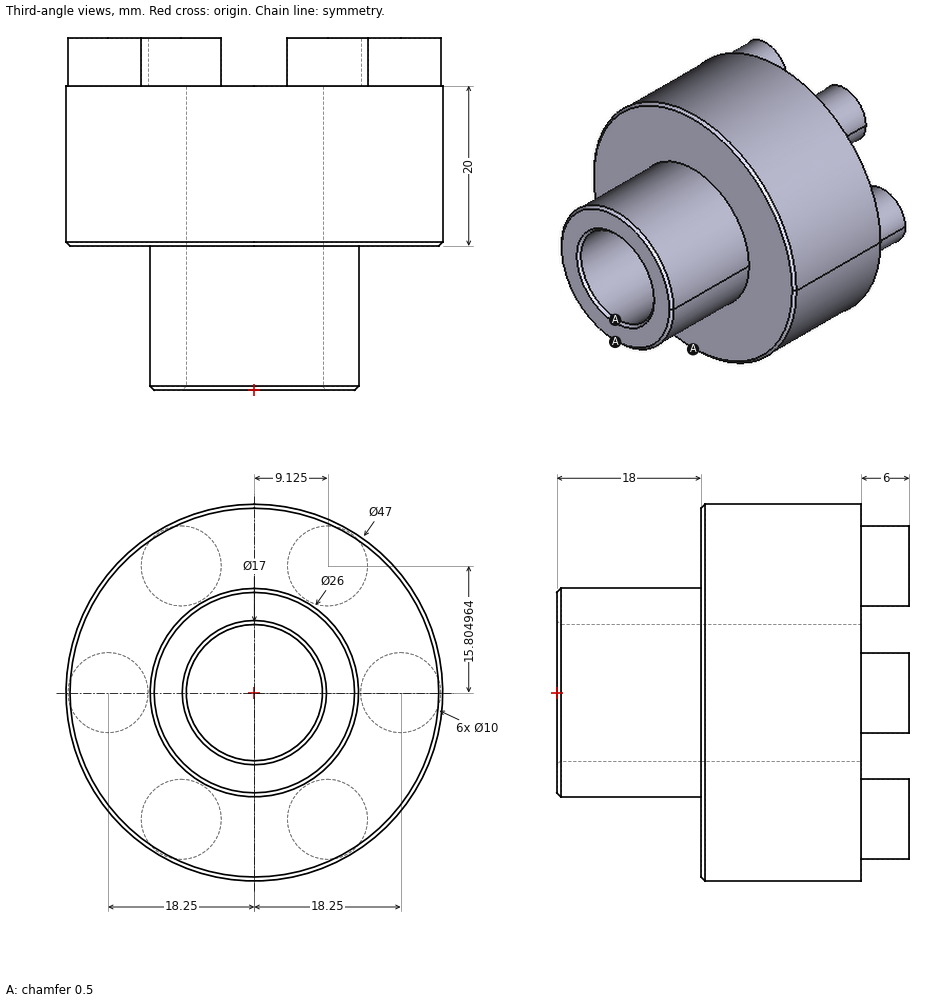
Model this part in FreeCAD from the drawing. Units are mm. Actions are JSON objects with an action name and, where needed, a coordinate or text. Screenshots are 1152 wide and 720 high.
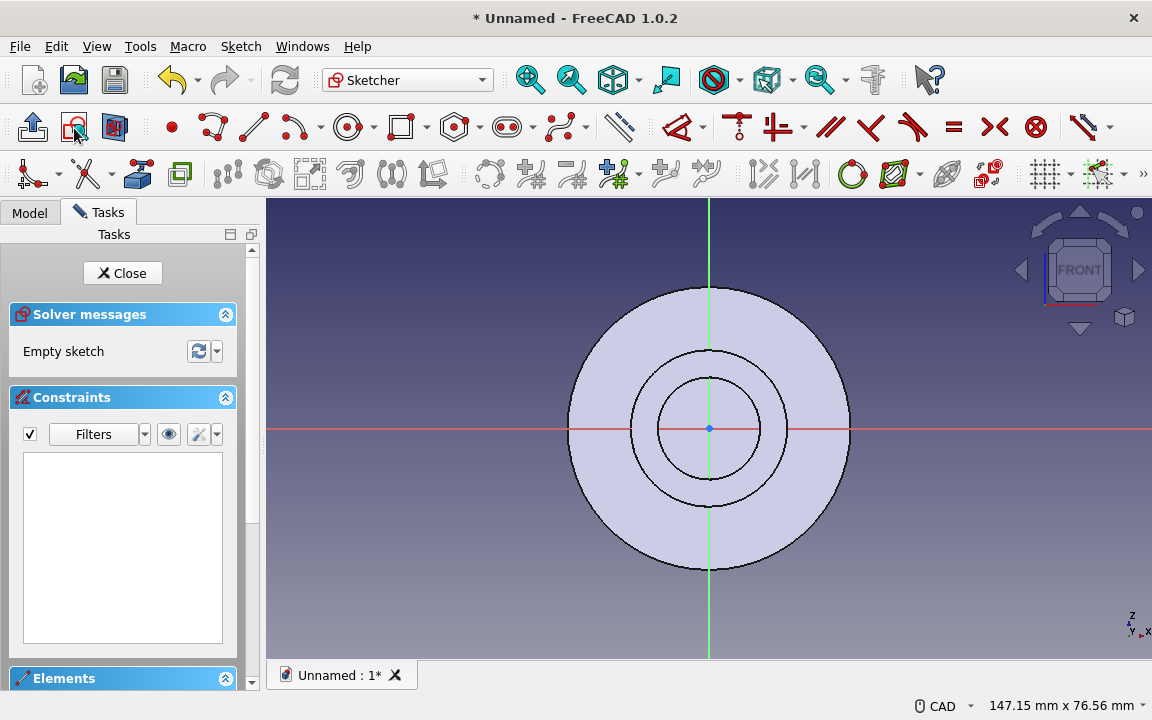
{"action": "left_click", "coordinate": [115, 128]}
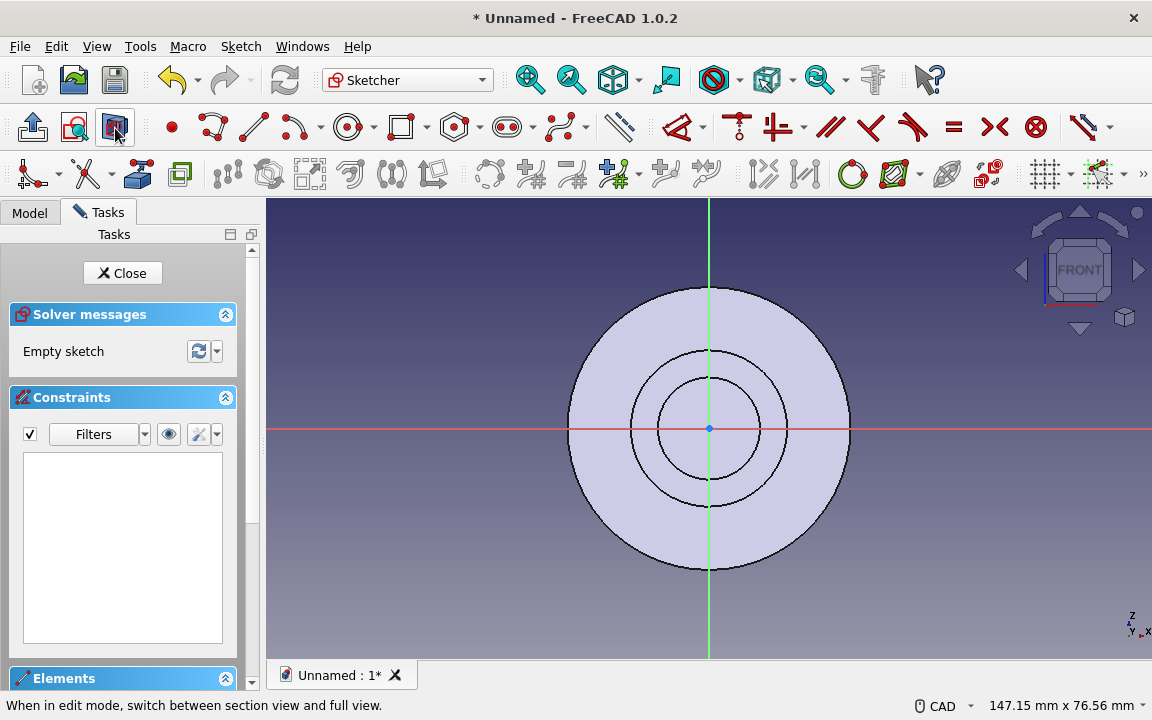
{"action": "scroll", "coordinate": [749, 429], "scroll_direction": "up", "scroll_amount": 5}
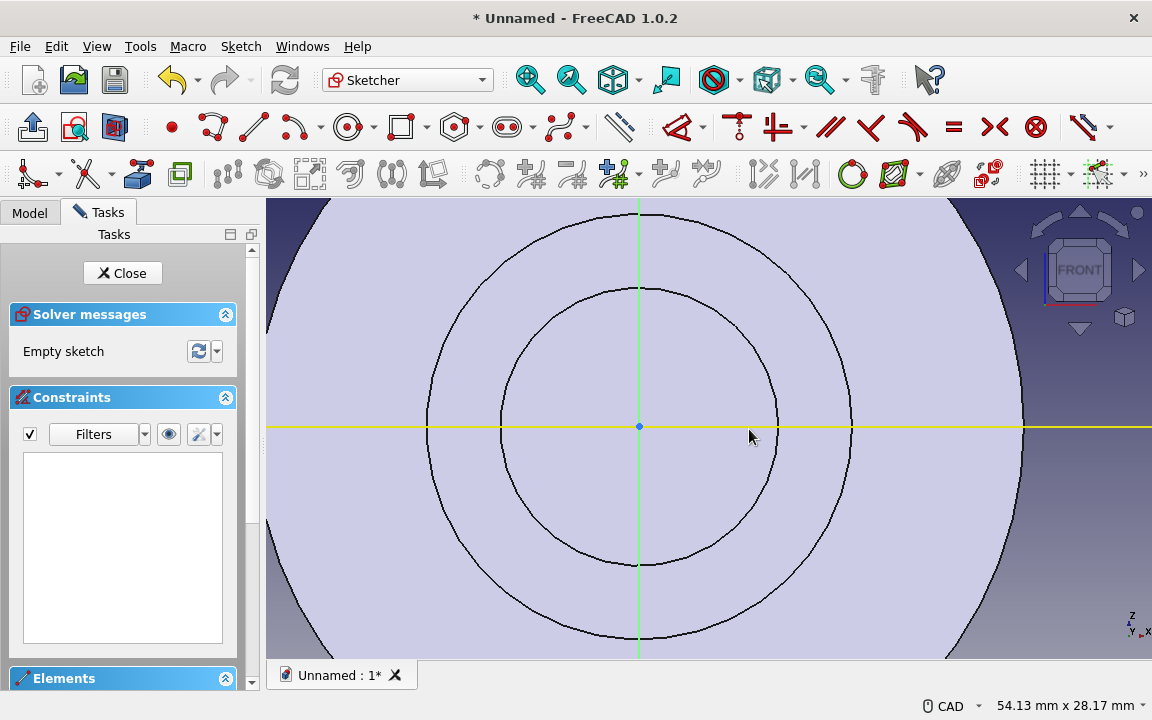
{"action": "left_click", "coordinate": [348, 128]}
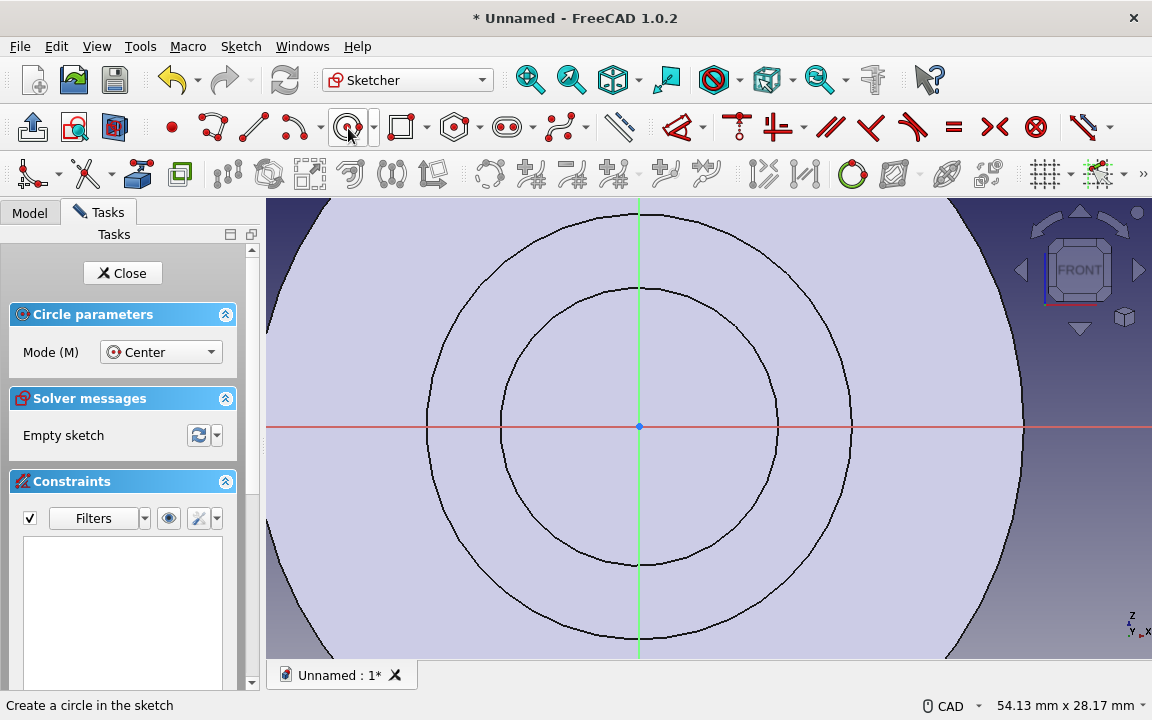
{"action": "left_click", "coordinate": [639, 427]}
{"action": "left_click", "coordinate": [738, 328]}
{"action": "key", "text": "Escape"}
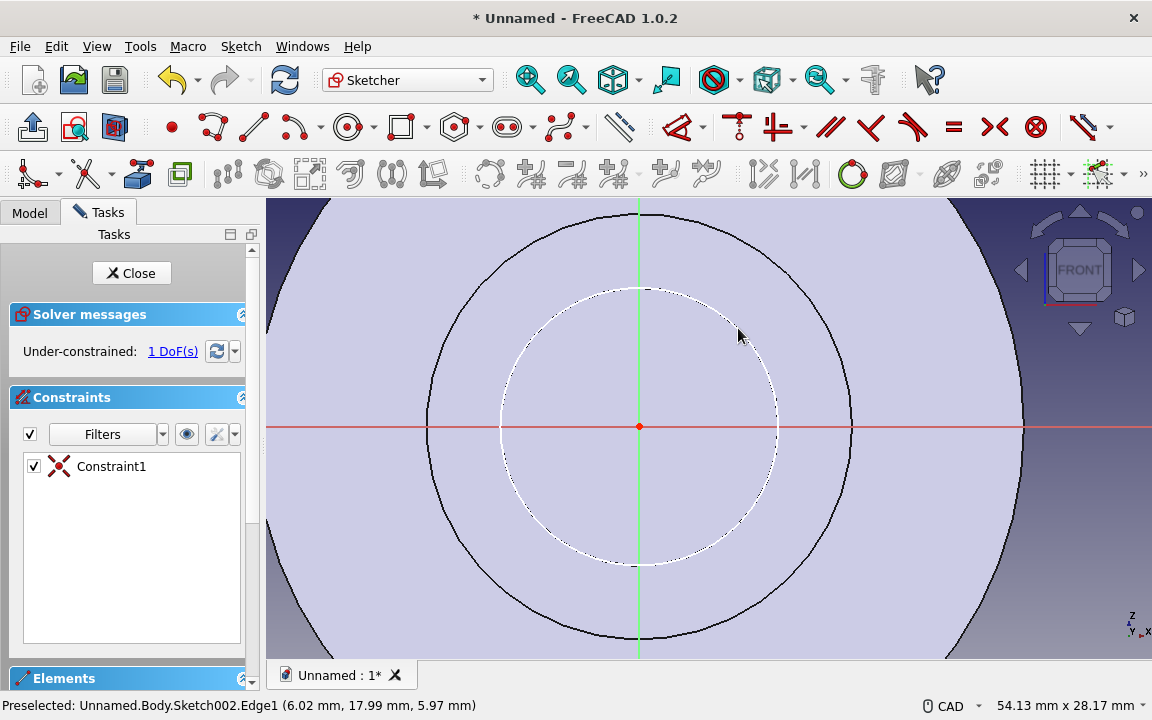
{"action": "left_click", "coordinate": [676, 128]}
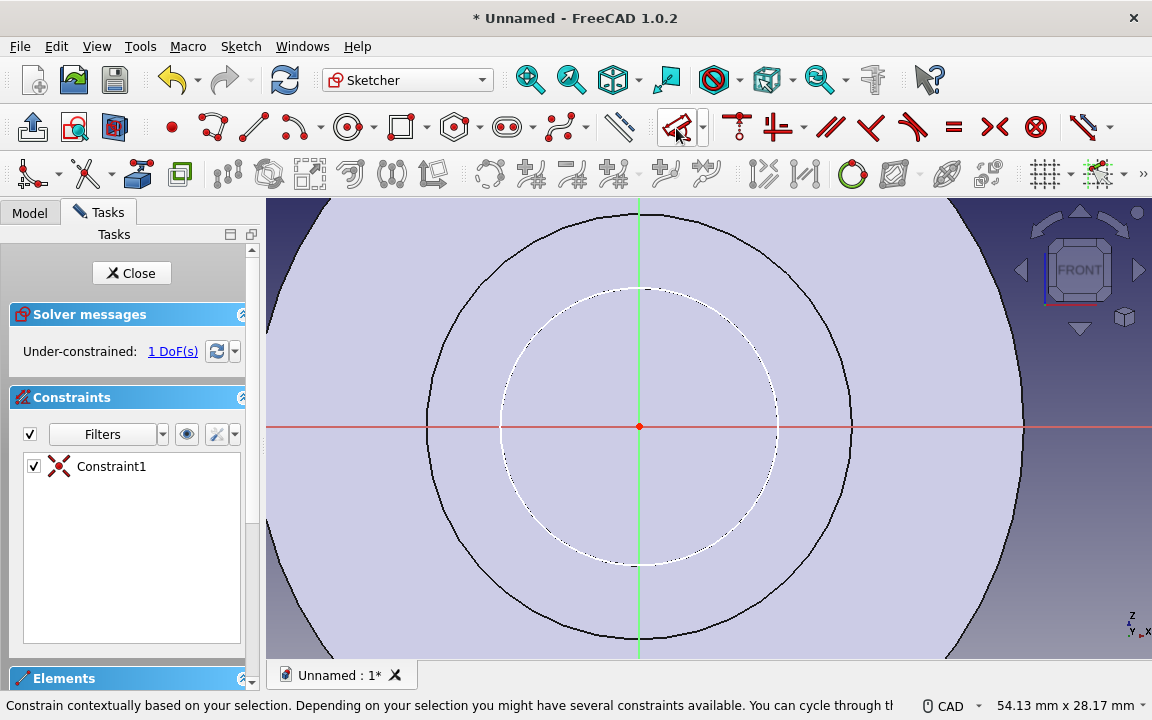
{"action": "left_click", "coordinate": [737, 328]}
{"action": "left_click", "coordinate": [759, 305]}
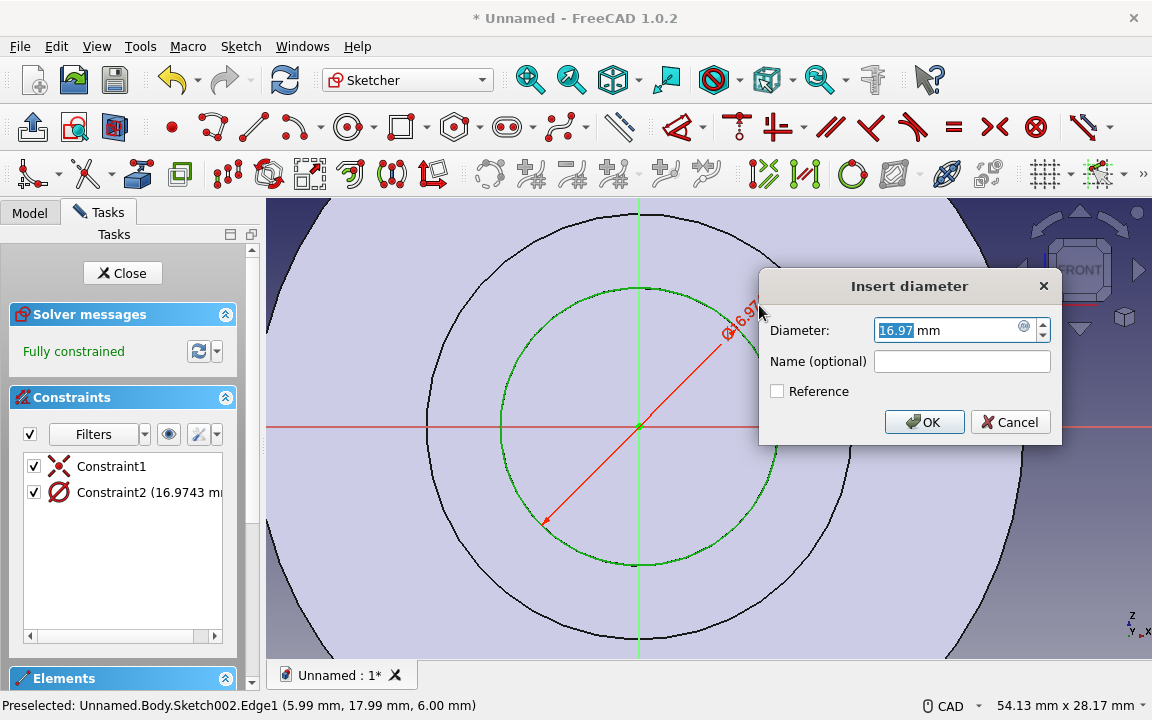
{"action": "type", "text": "17"}
{"action": "key", "text": "Return"}
{"action": "key", "text": "Escape"}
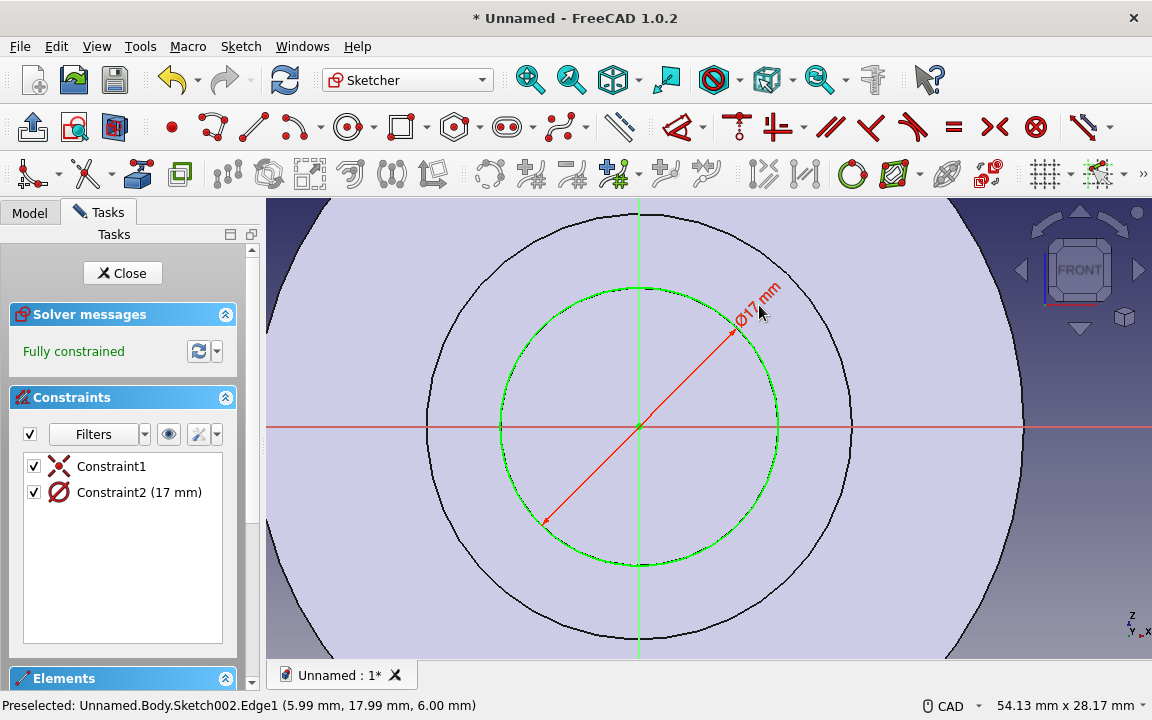
{"action": "left_click", "coordinate": [123, 273]}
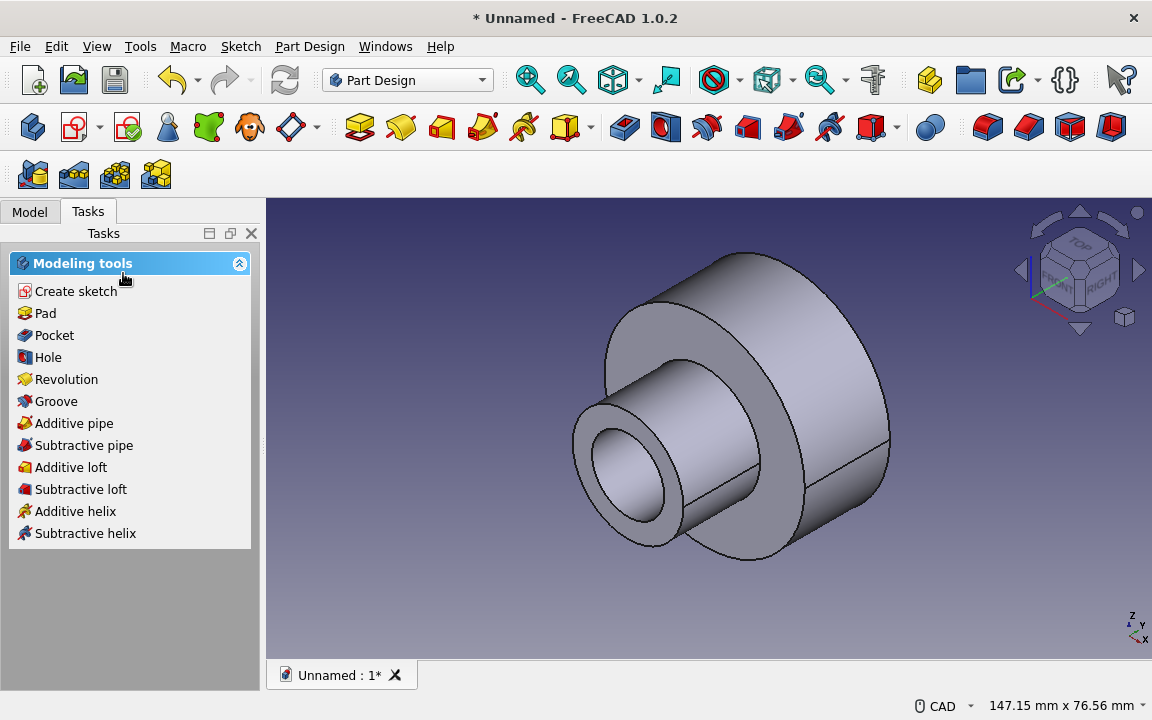
{"action": "left_click", "coordinate": [625, 128]}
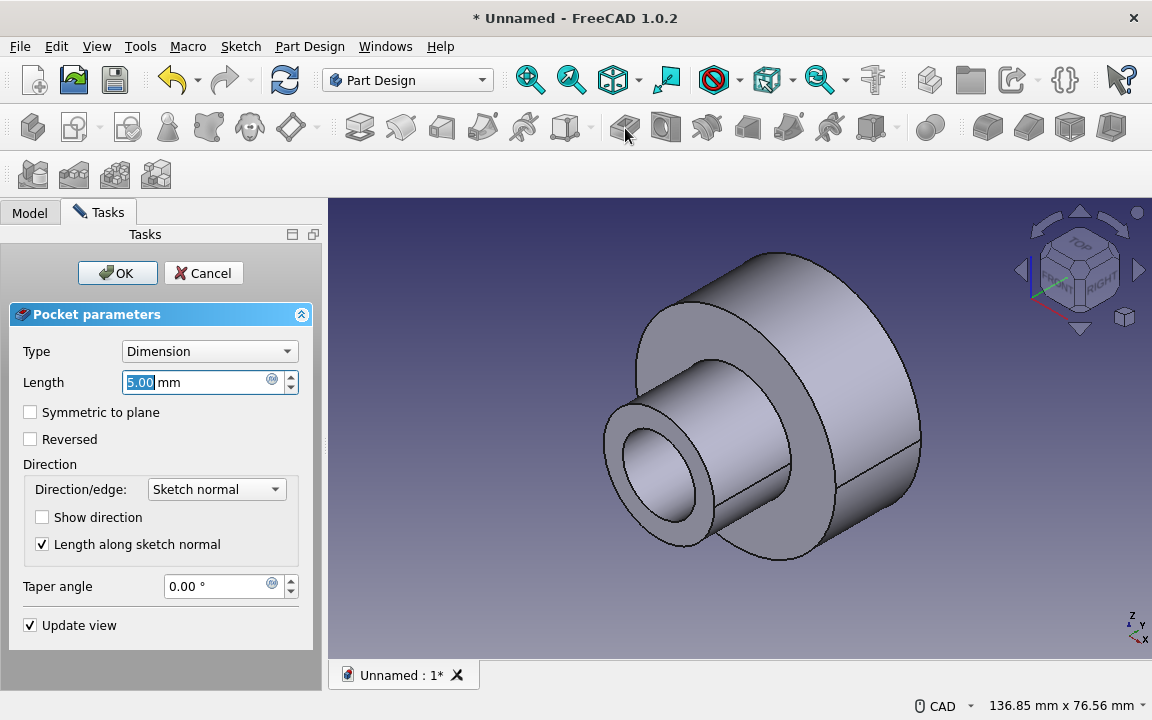
{"action": "left_click", "coordinate": [210, 352]}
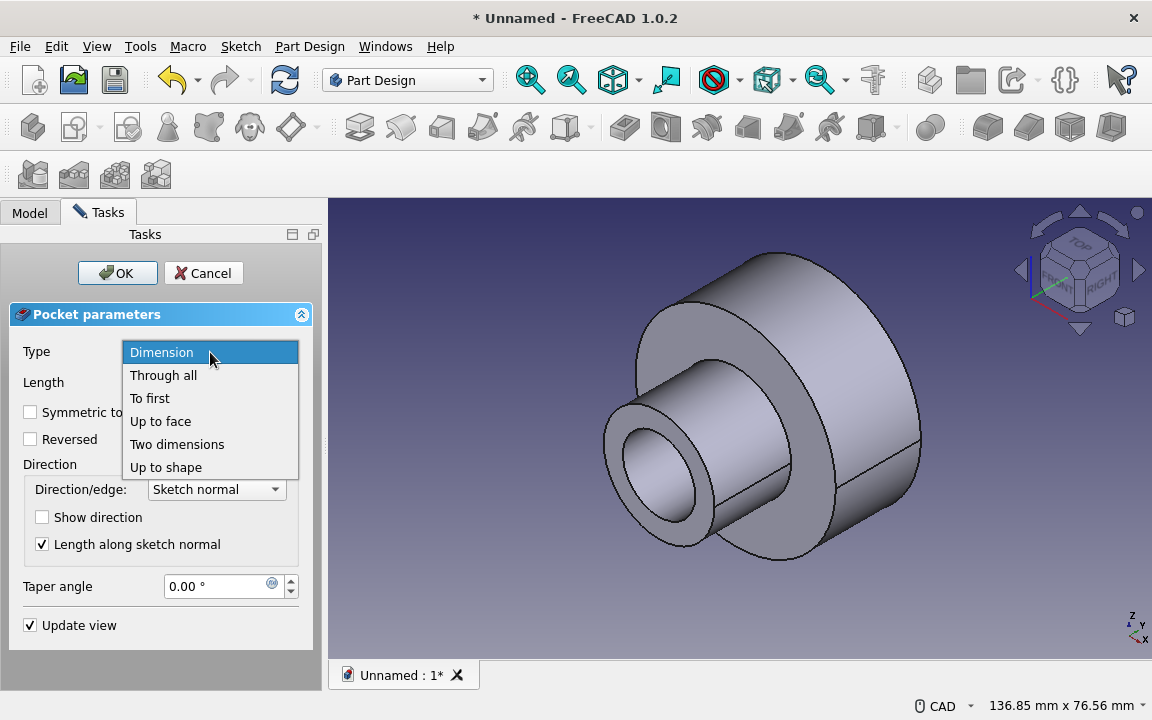
{"action": "left_click", "coordinate": [208, 376]}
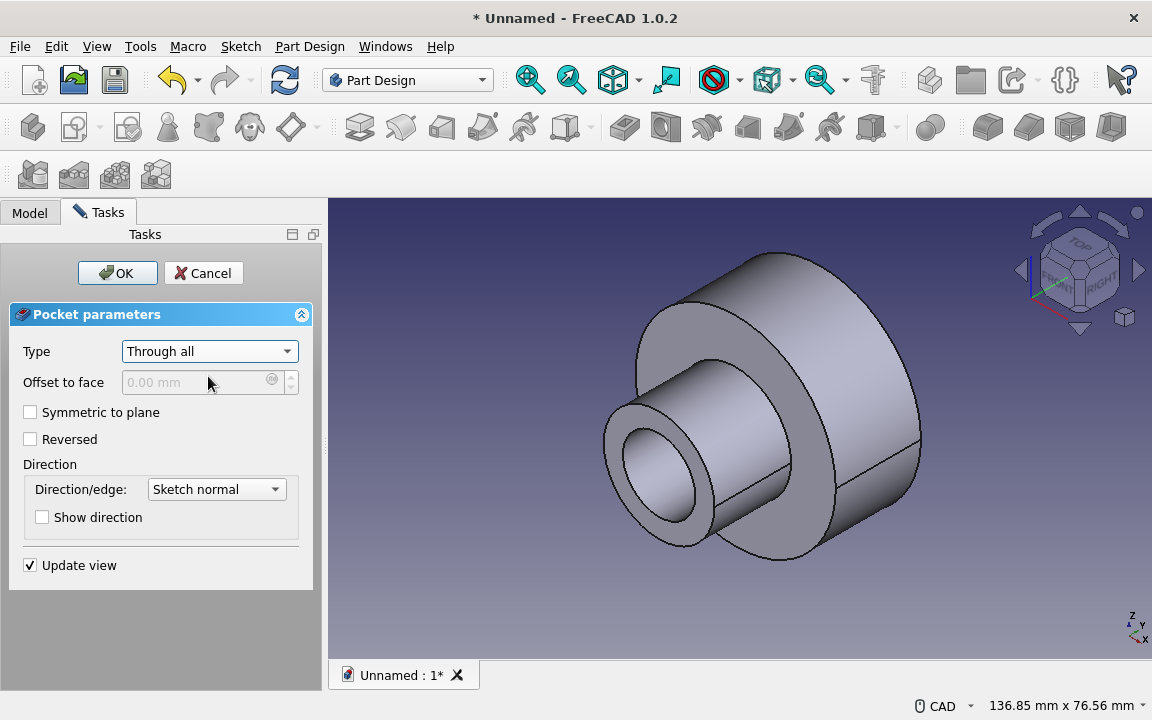
{"action": "left_click", "coordinate": [118, 273]}